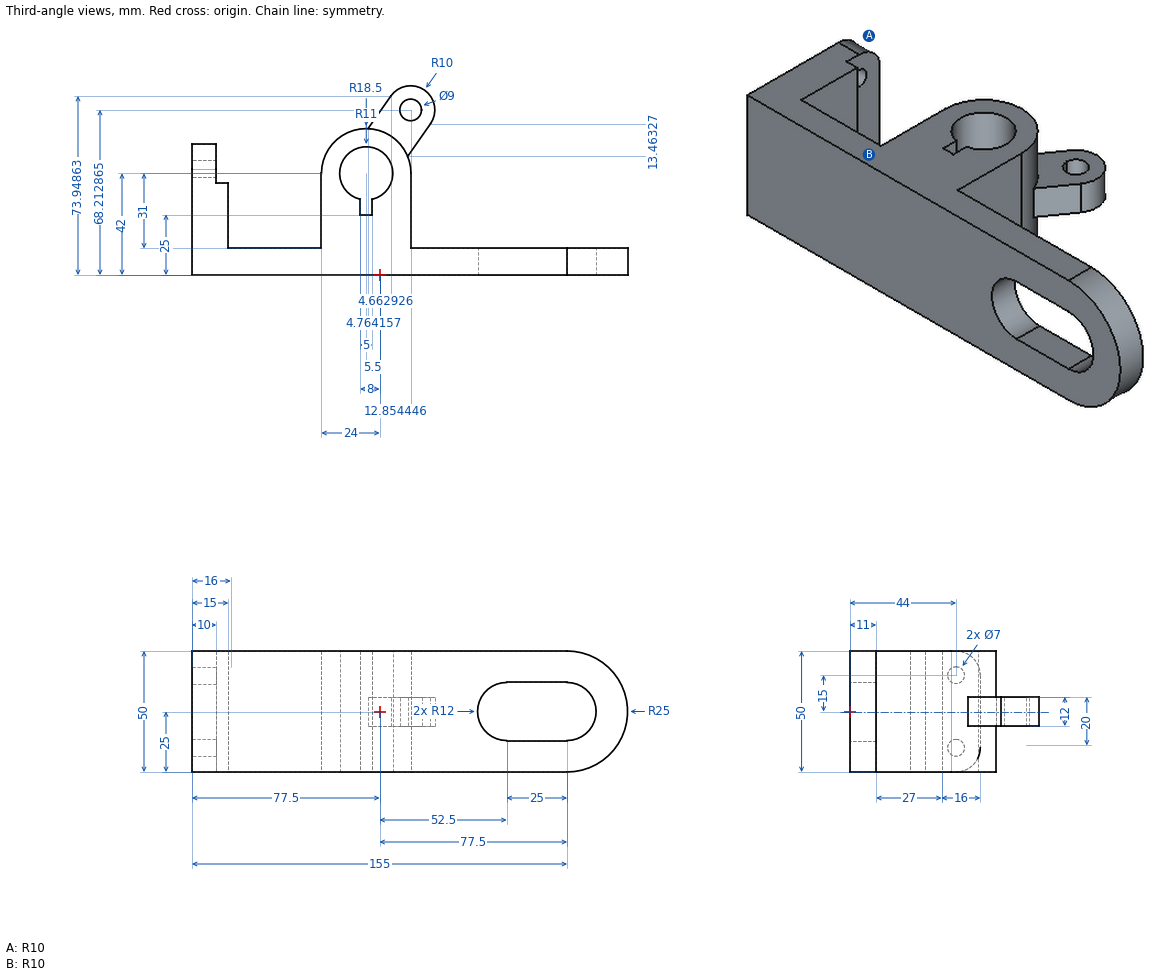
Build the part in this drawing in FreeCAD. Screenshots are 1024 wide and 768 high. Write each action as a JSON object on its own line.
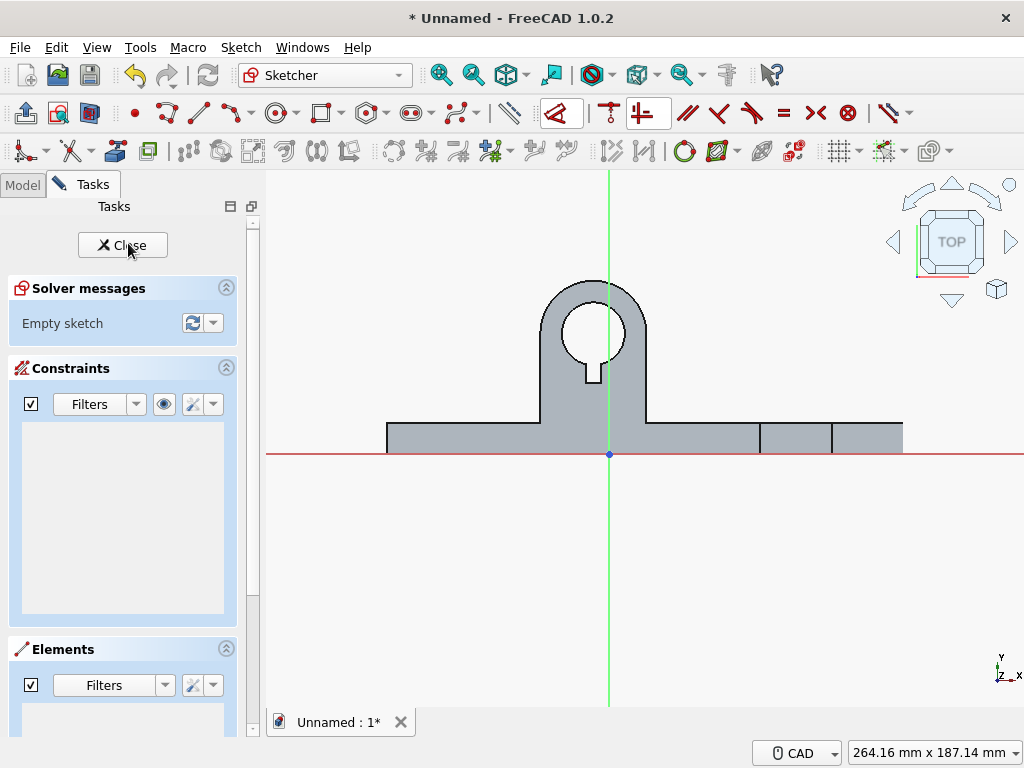
{"action": "scroll", "coordinate": [651, 221], "scroll_direction": "up", "scroll_amount": 7}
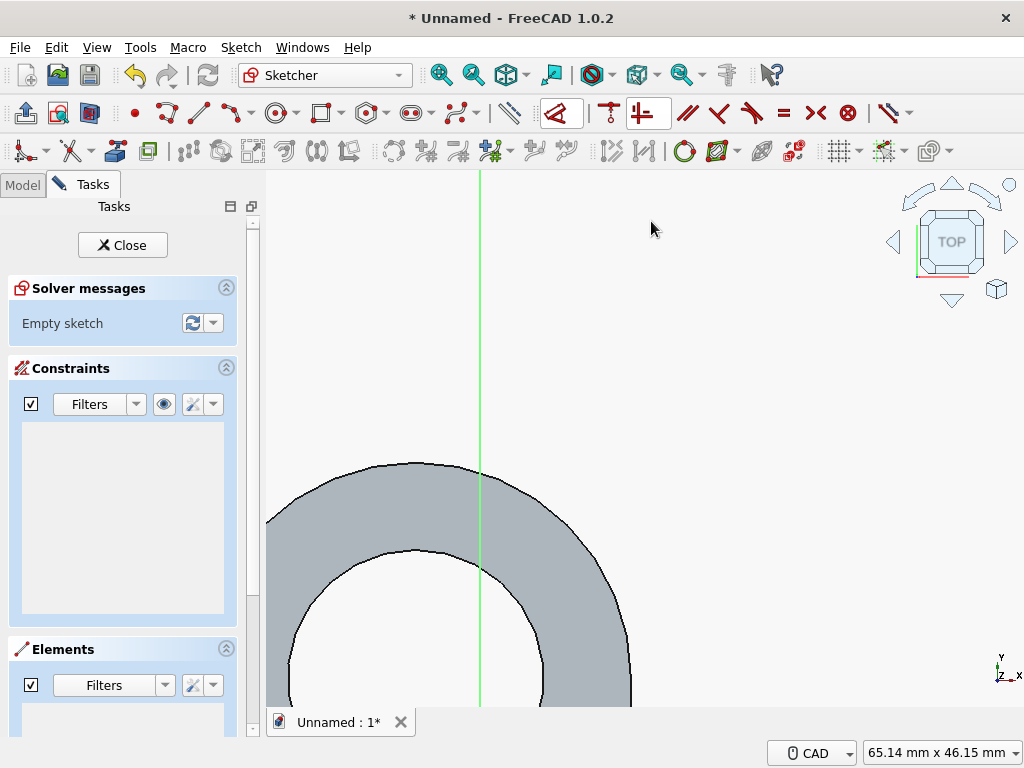
{"action": "left_click", "coordinate": [200, 114]}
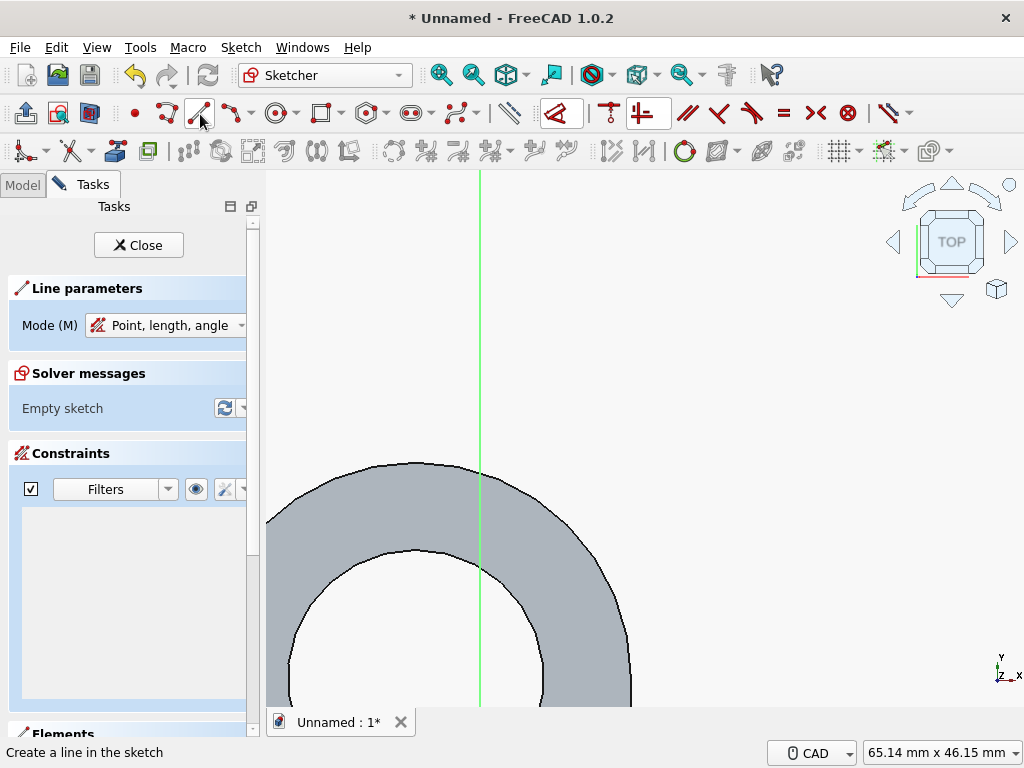
{"action": "left_click", "coordinate": [615, 596]}
{"action": "left_click", "coordinate": [725, 440]}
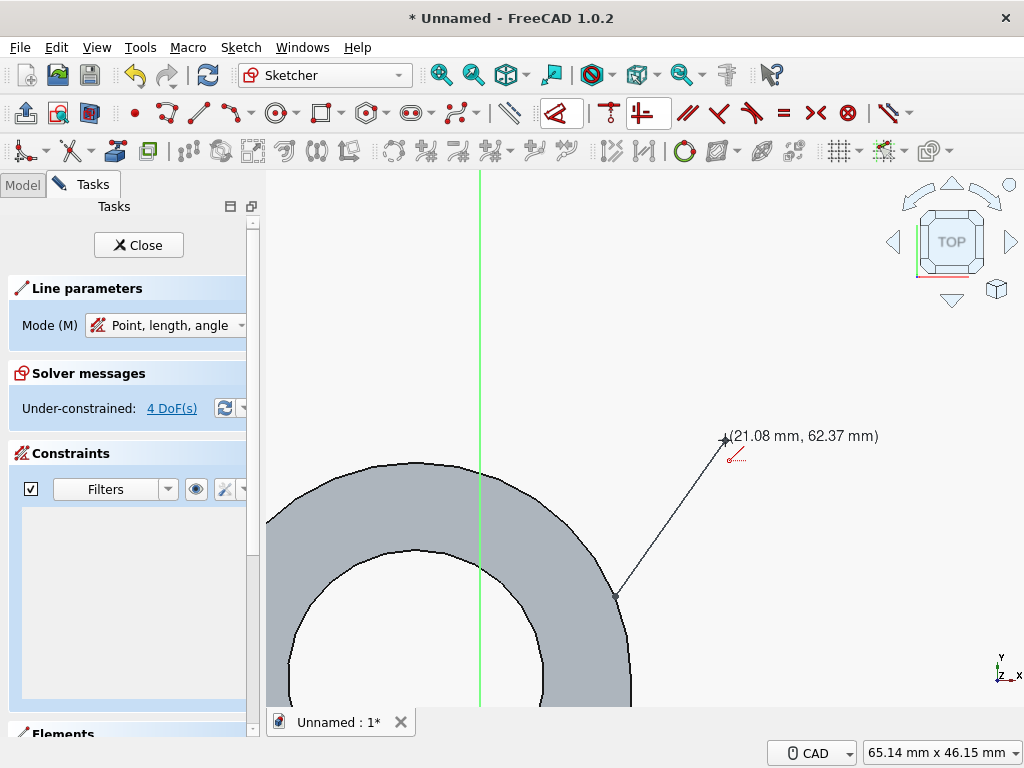
{"action": "left_click", "coordinate": [534, 306]}
{"action": "left_click", "coordinate": [424, 463]}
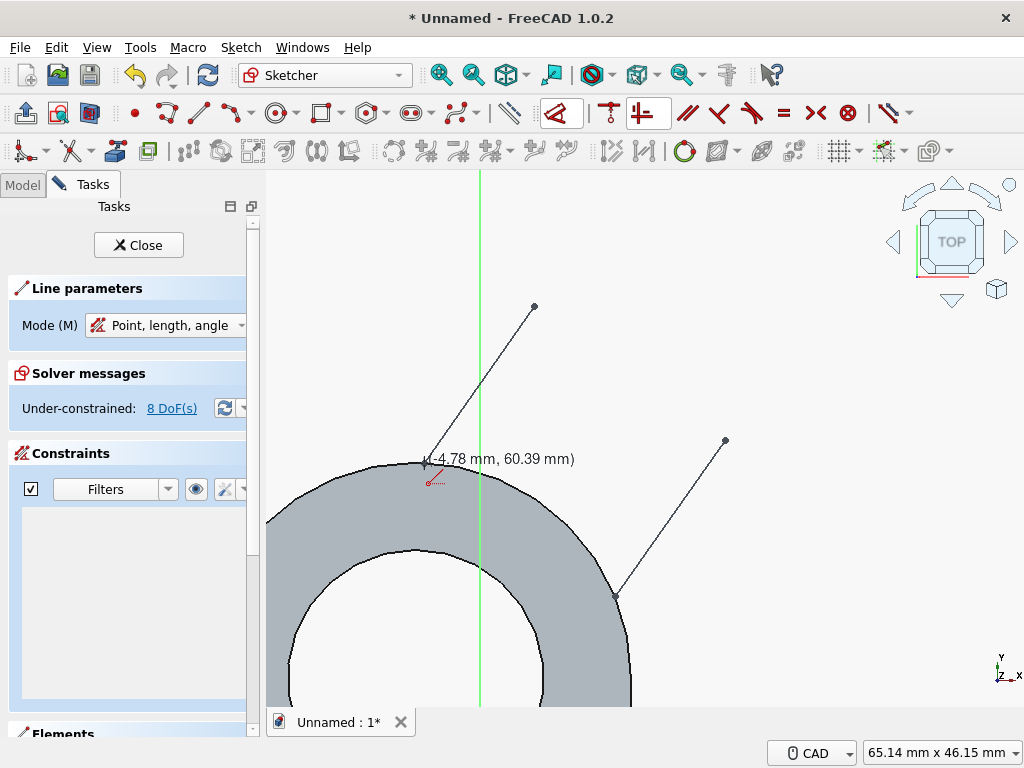
{"action": "left_click", "coordinate": [232, 114]}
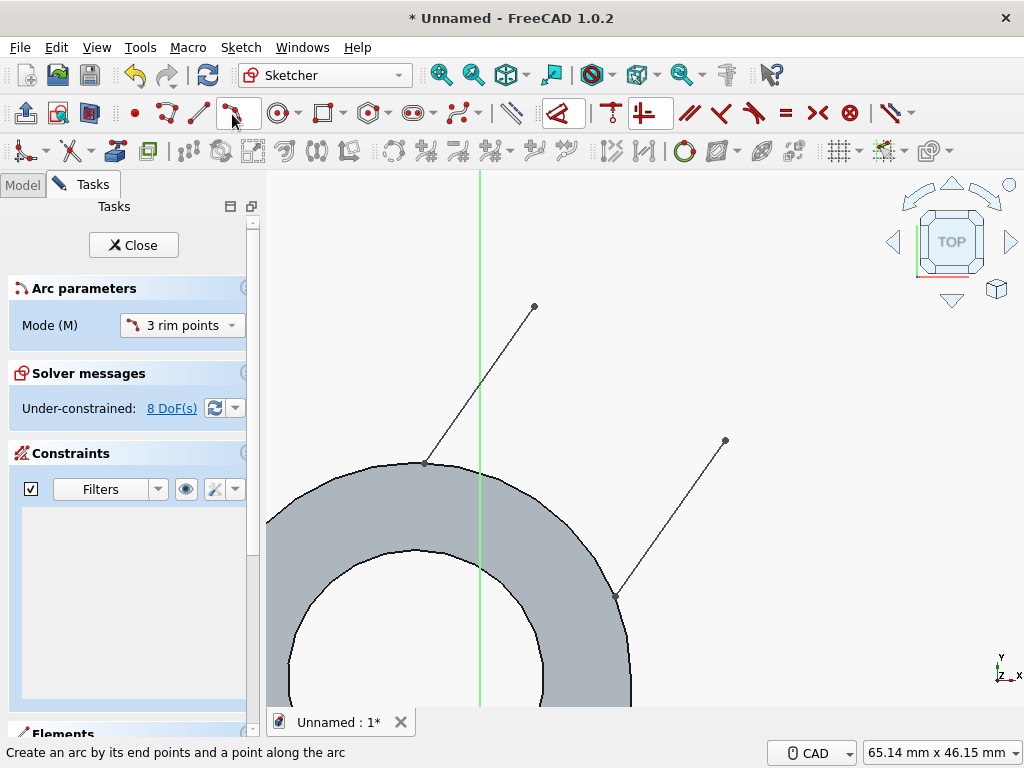
{"action": "left_click", "coordinate": [725, 441]}
{"action": "left_click", "coordinate": [534, 307]}
{"action": "left_click", "coordinate": [696, 278]}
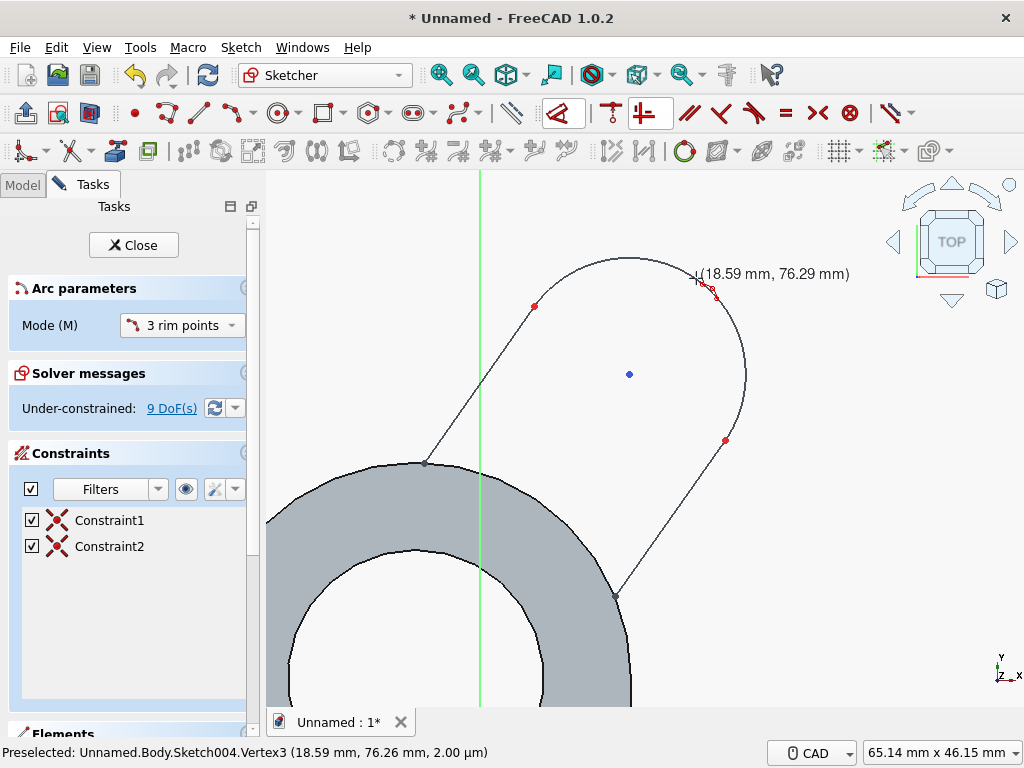
{"action": "left_click", "coordinate": [424, 464]}
{"action": "left_click", "coordinate": [615, 597]}
{"action": "left_click", "coordinate": [539, 502]}
{"action": "key", "text": "Escape"}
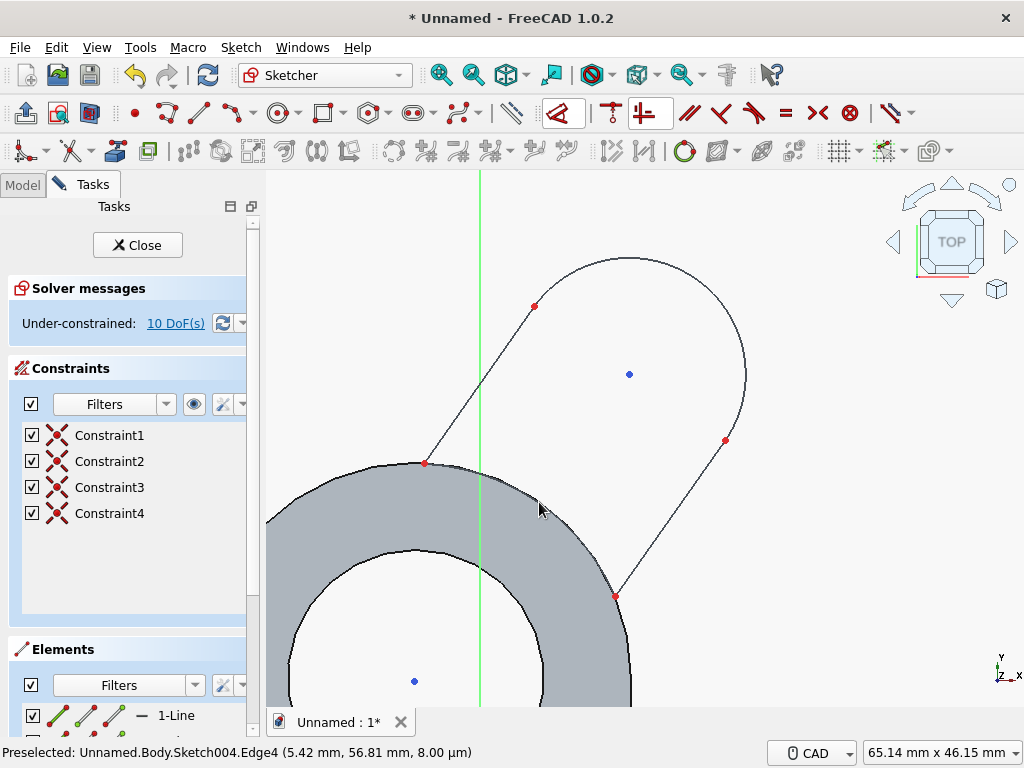
{"action": "left_click", "coordinate": [648, 550]}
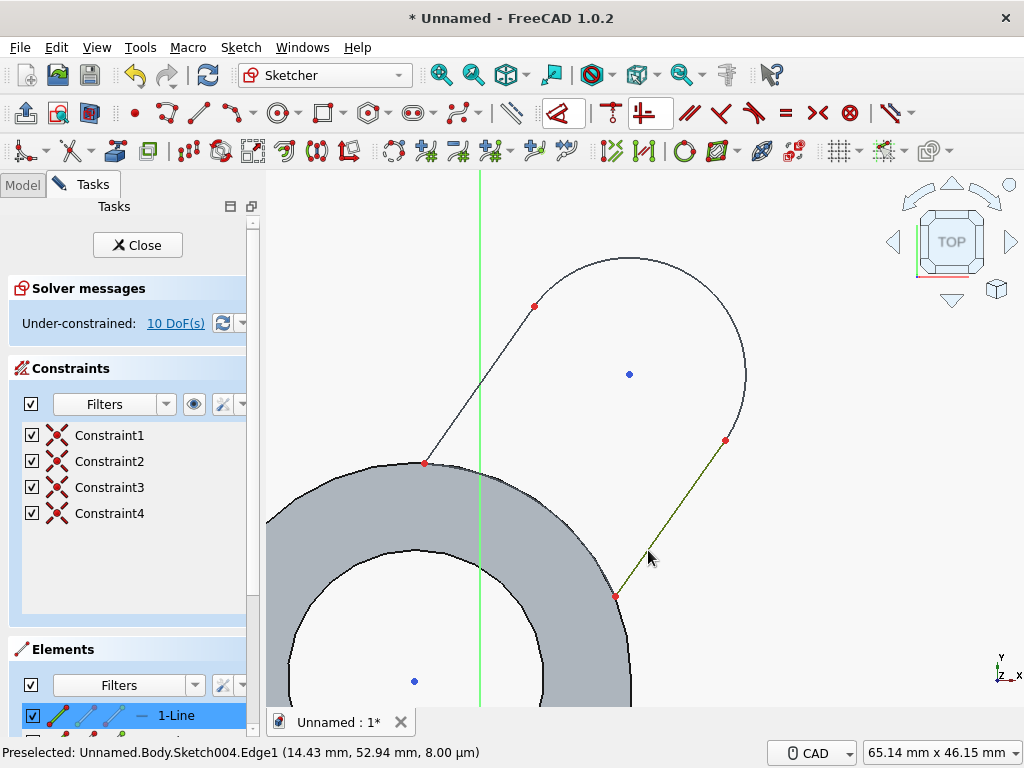
{"action": "left_click", "coordinate": [739, 336]}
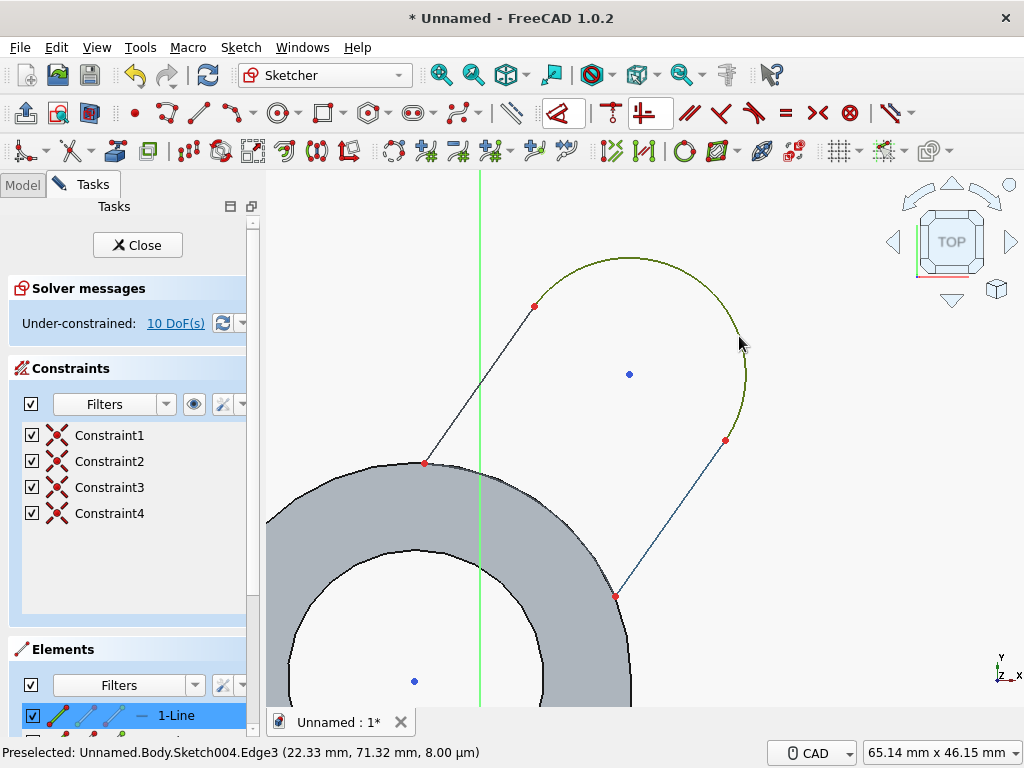
{"action": "key", "text": "t"}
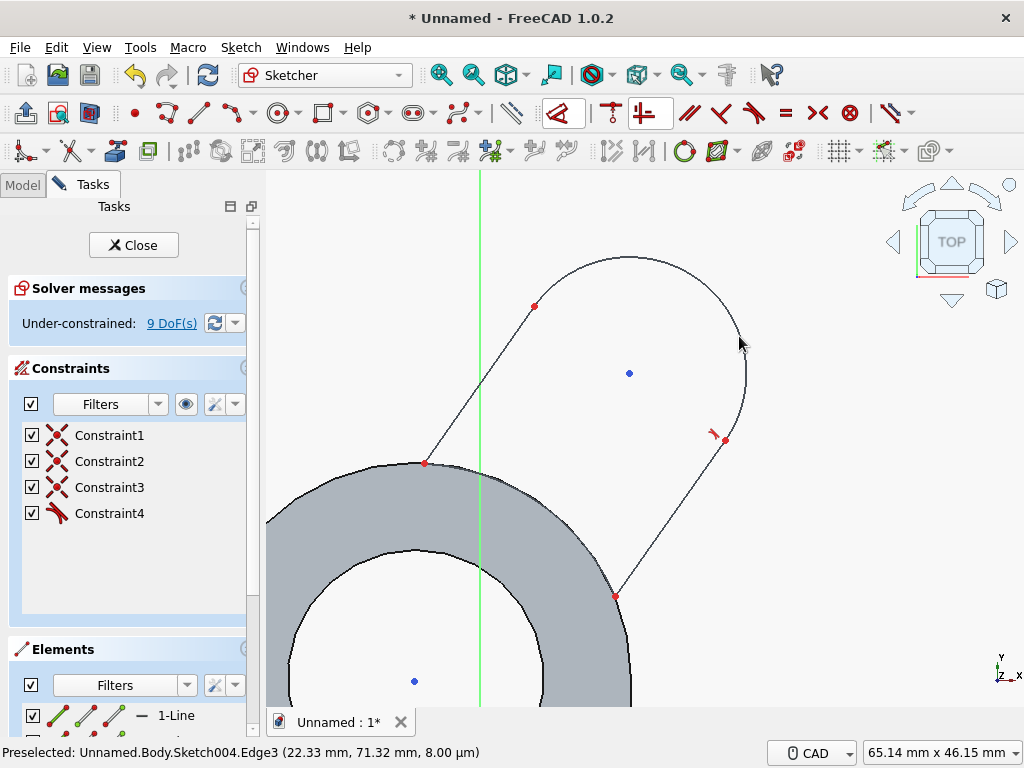
{"action": "left_click", "coordinate": [501, 354]}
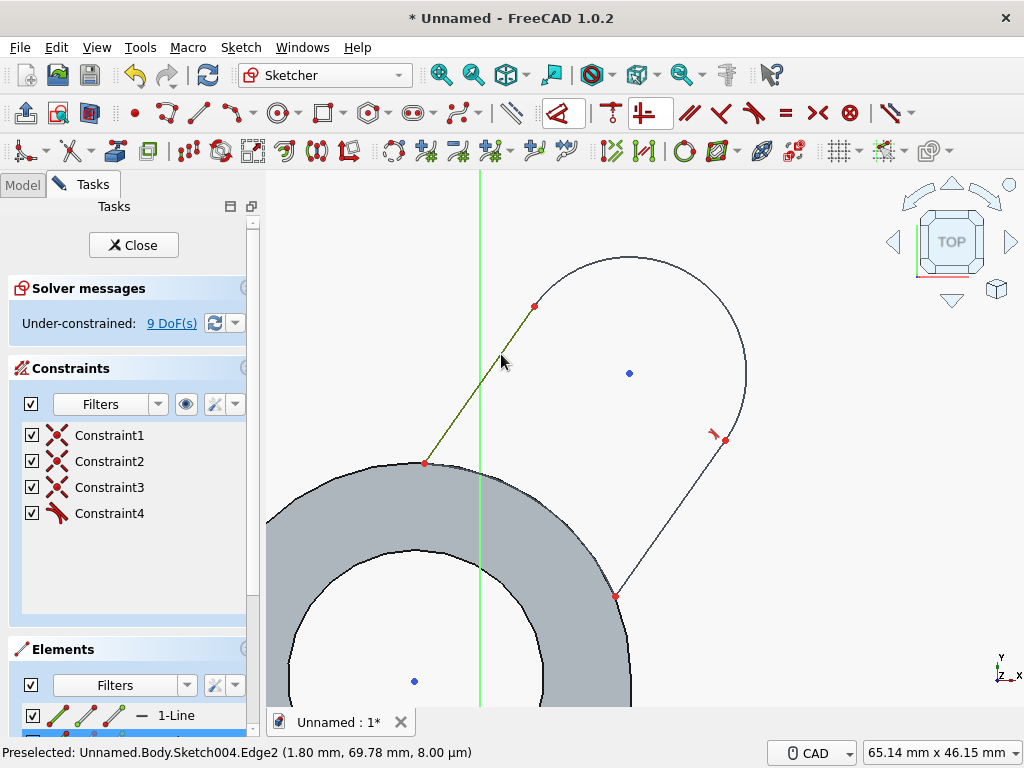
{"action": "left_click", "coordinate": [740, 336]}